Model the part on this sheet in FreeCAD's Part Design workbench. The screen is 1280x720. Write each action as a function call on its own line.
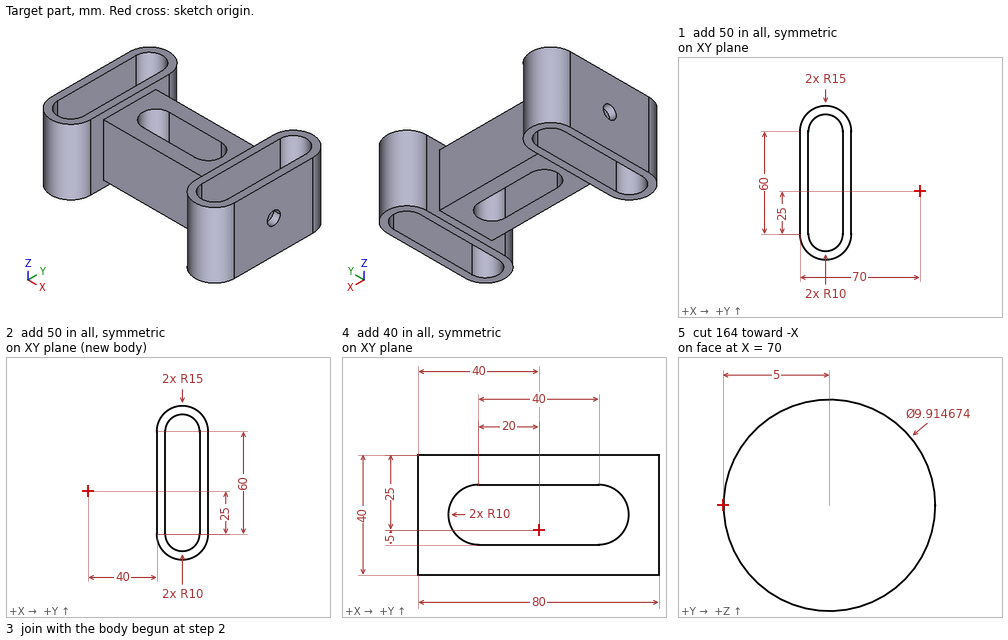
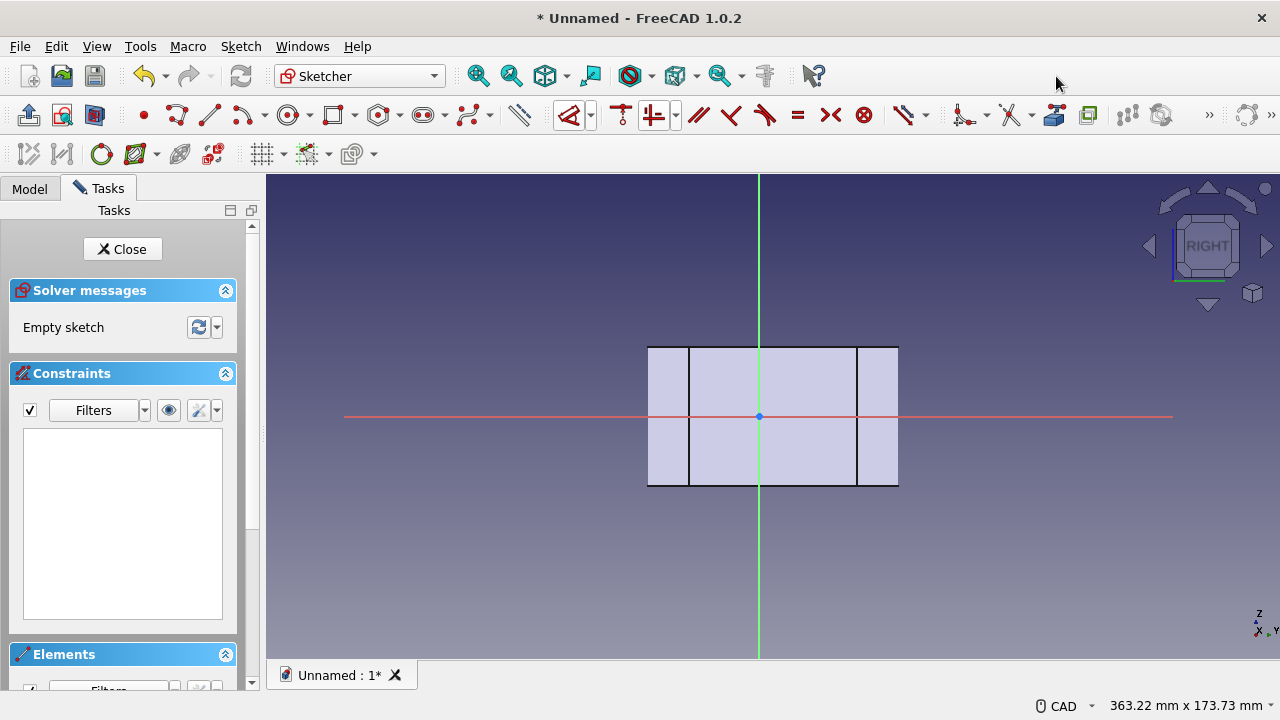
scroll(780, 416, up, 12)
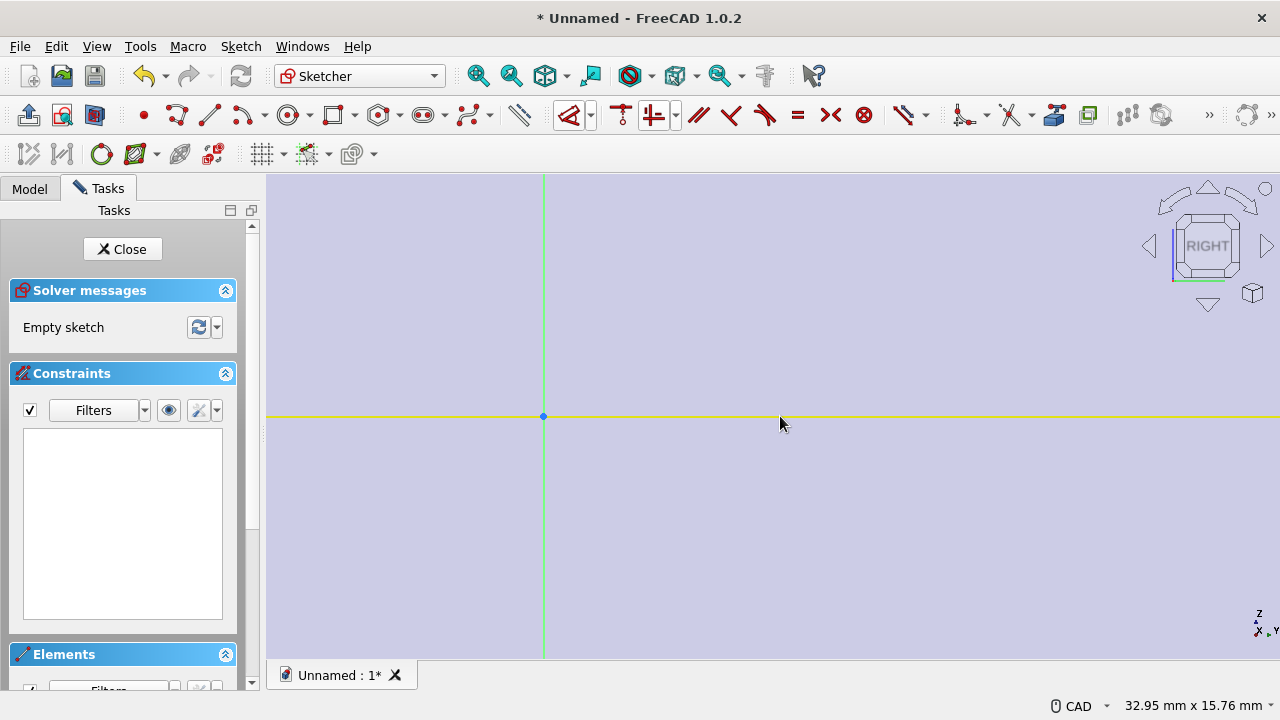
click(288, 116)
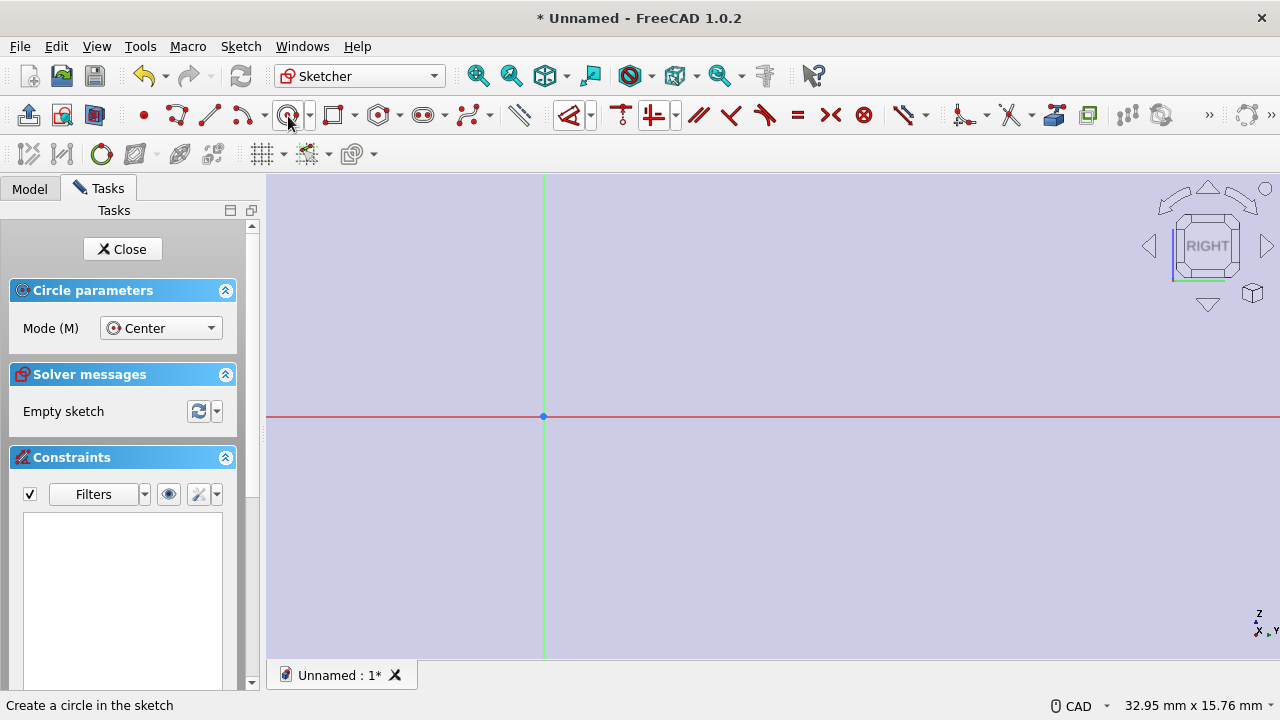
click(698, 416)
click(806, 309)
key(Escape)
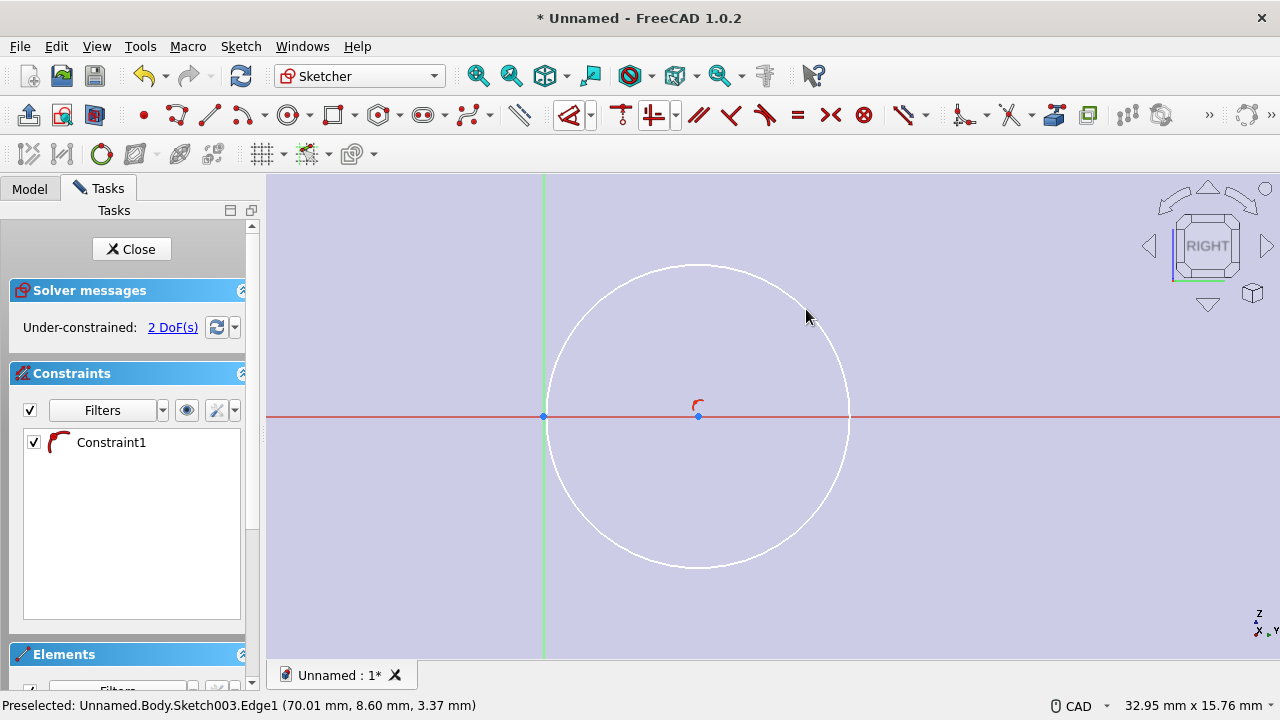
click(805, 309)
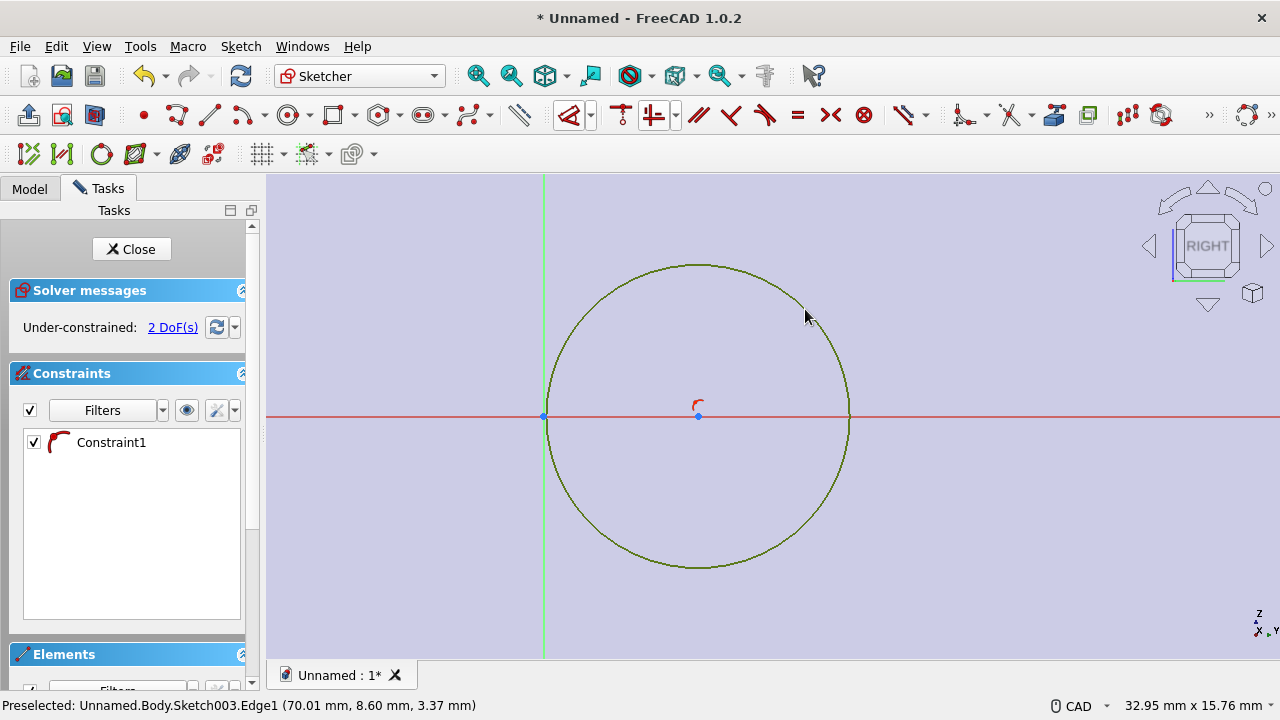
click(590, 116)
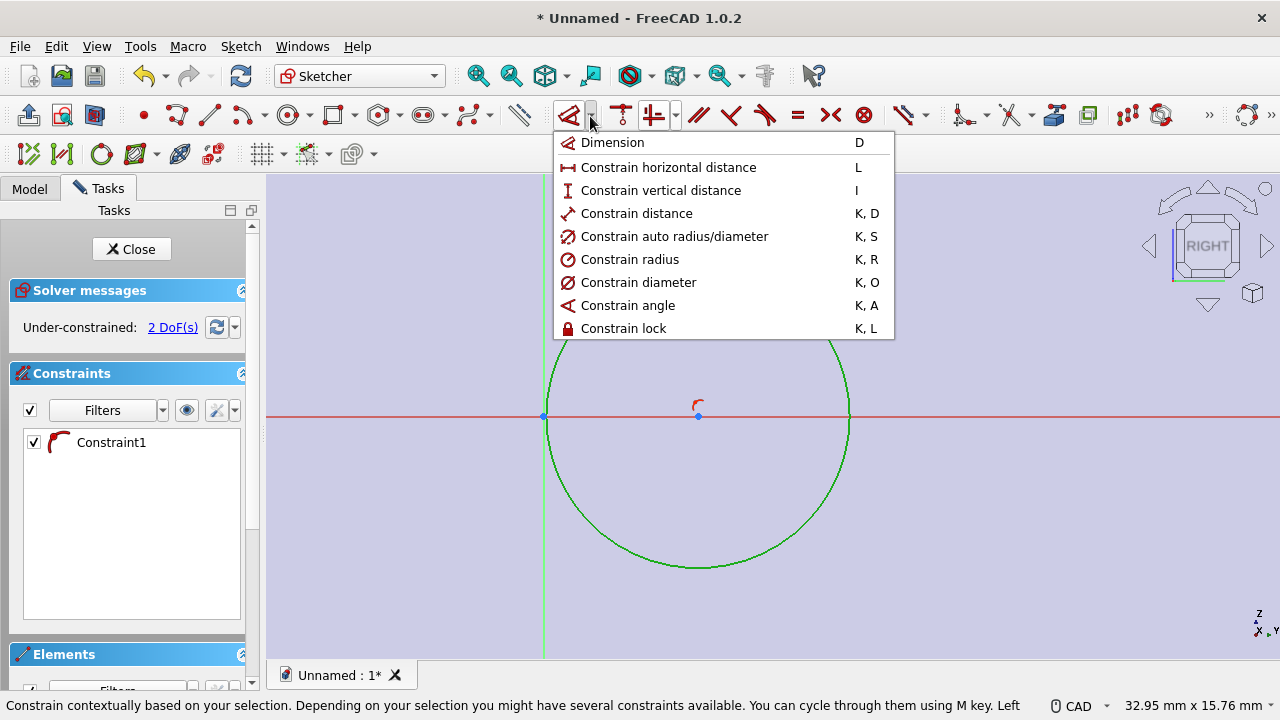
click(724, 282)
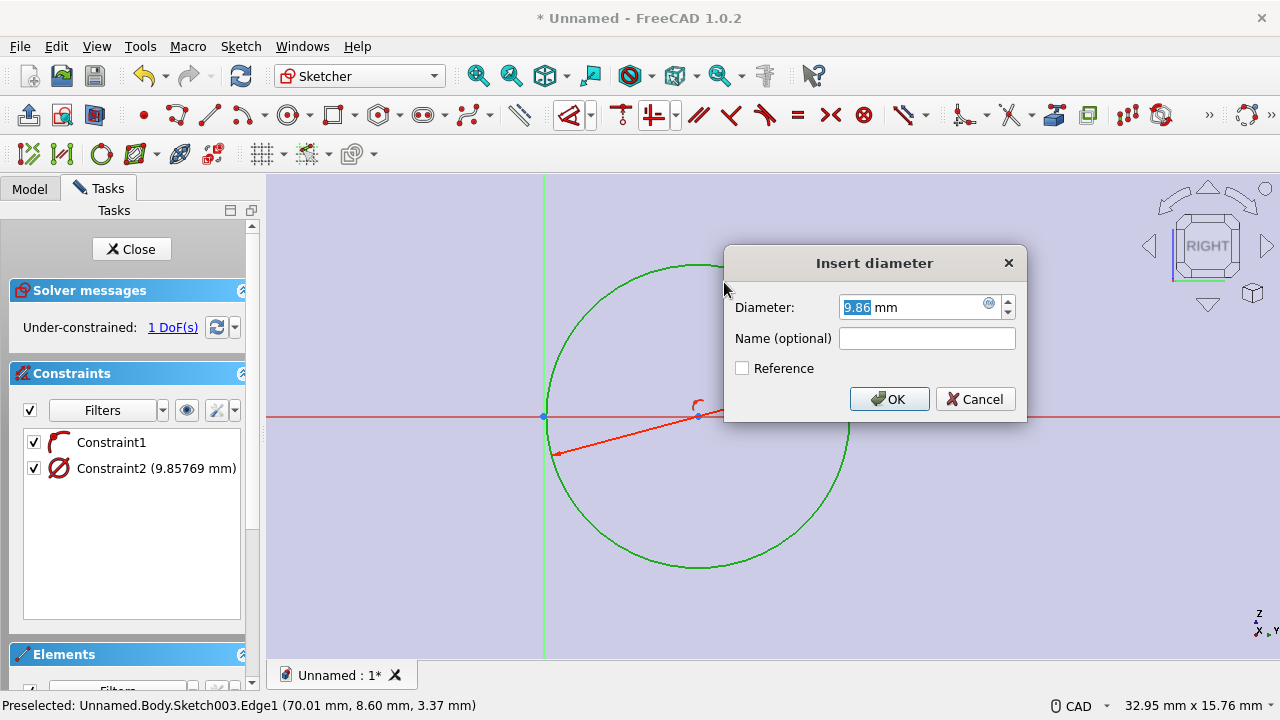
text(9.914674)
key(Return)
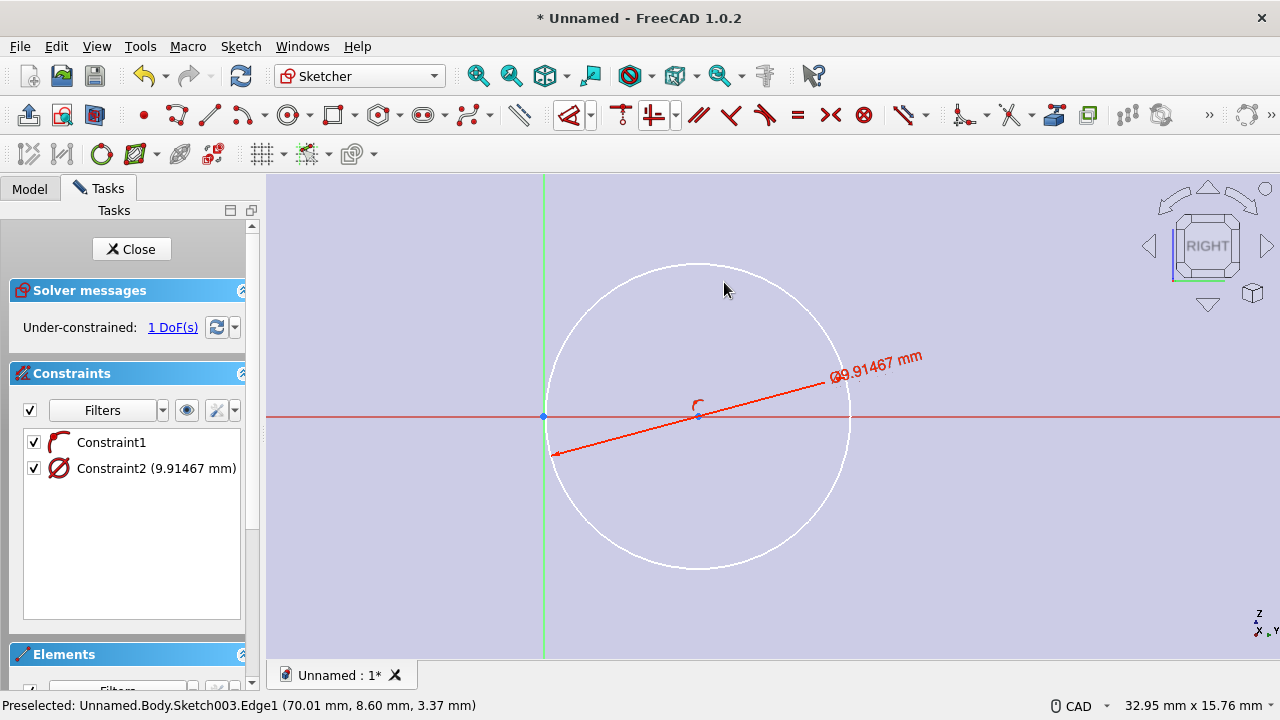
click(698, 416)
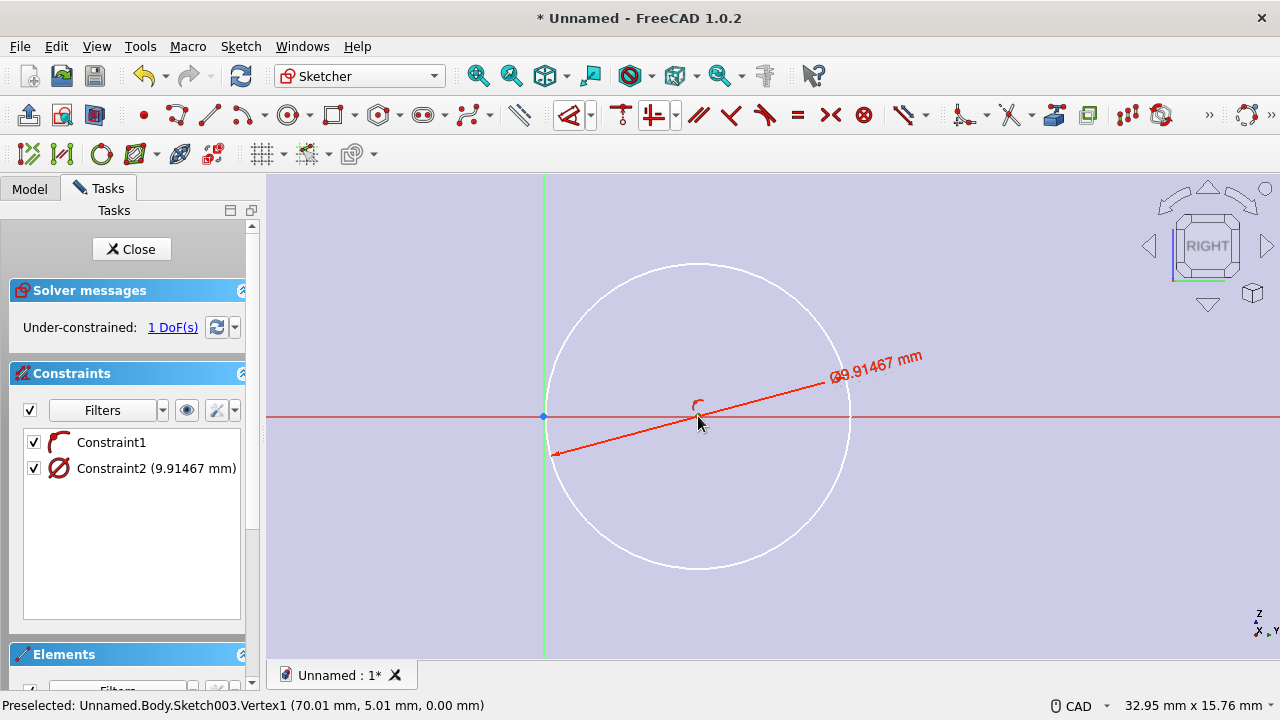
click(590, 116)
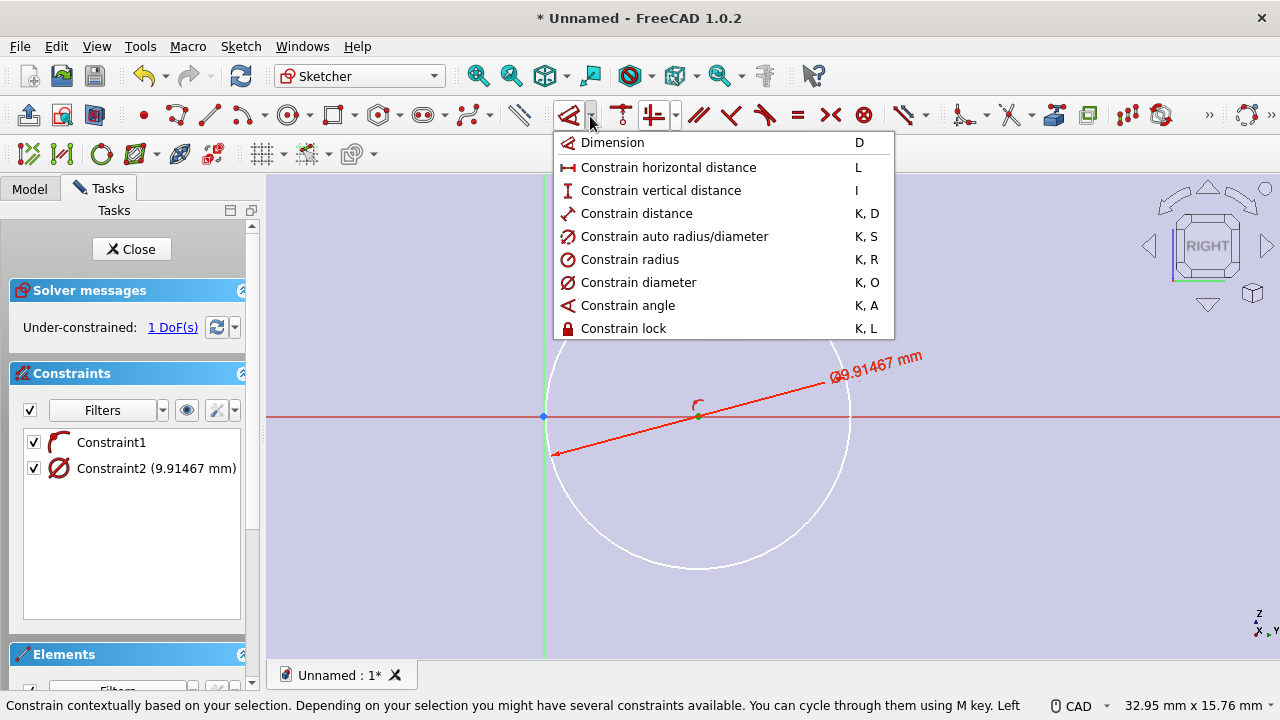
click(724, 168)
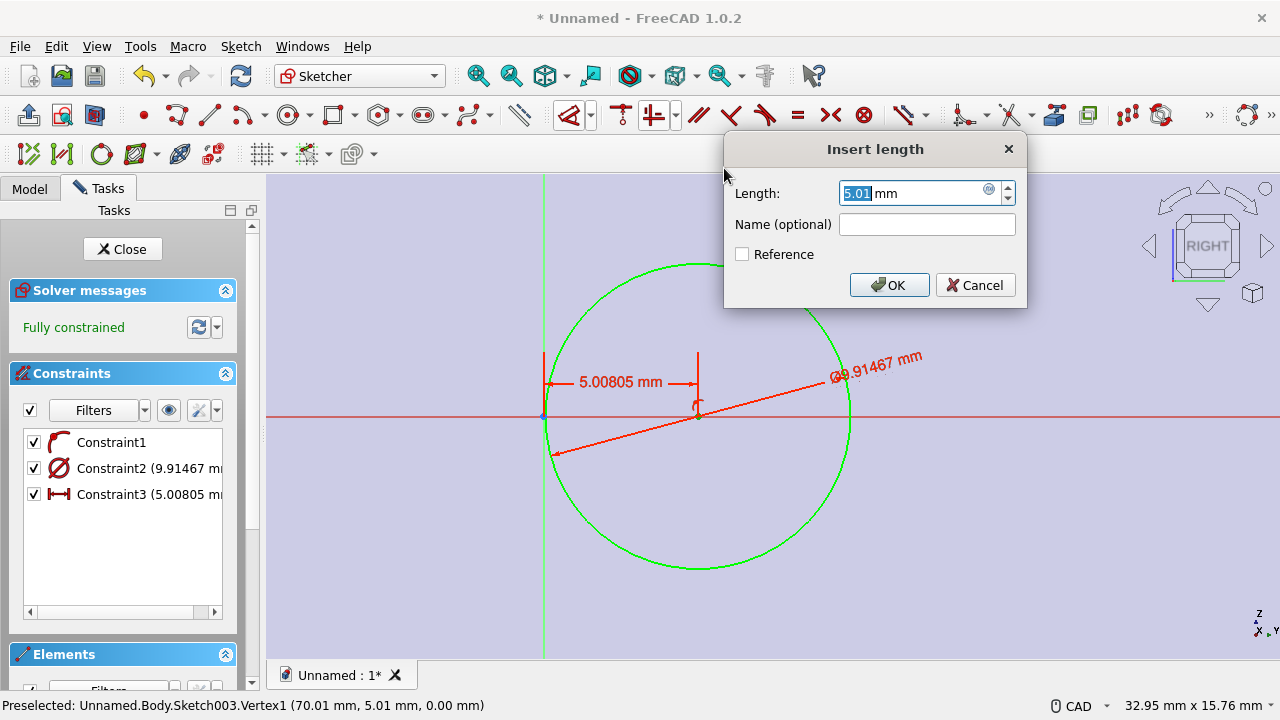
text(5)
key(Return)